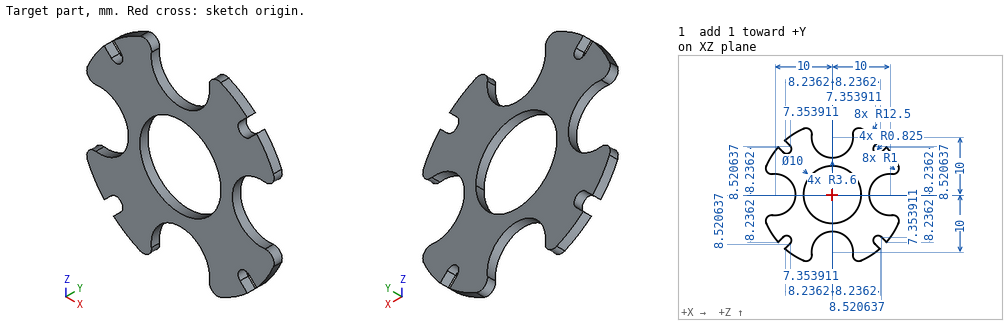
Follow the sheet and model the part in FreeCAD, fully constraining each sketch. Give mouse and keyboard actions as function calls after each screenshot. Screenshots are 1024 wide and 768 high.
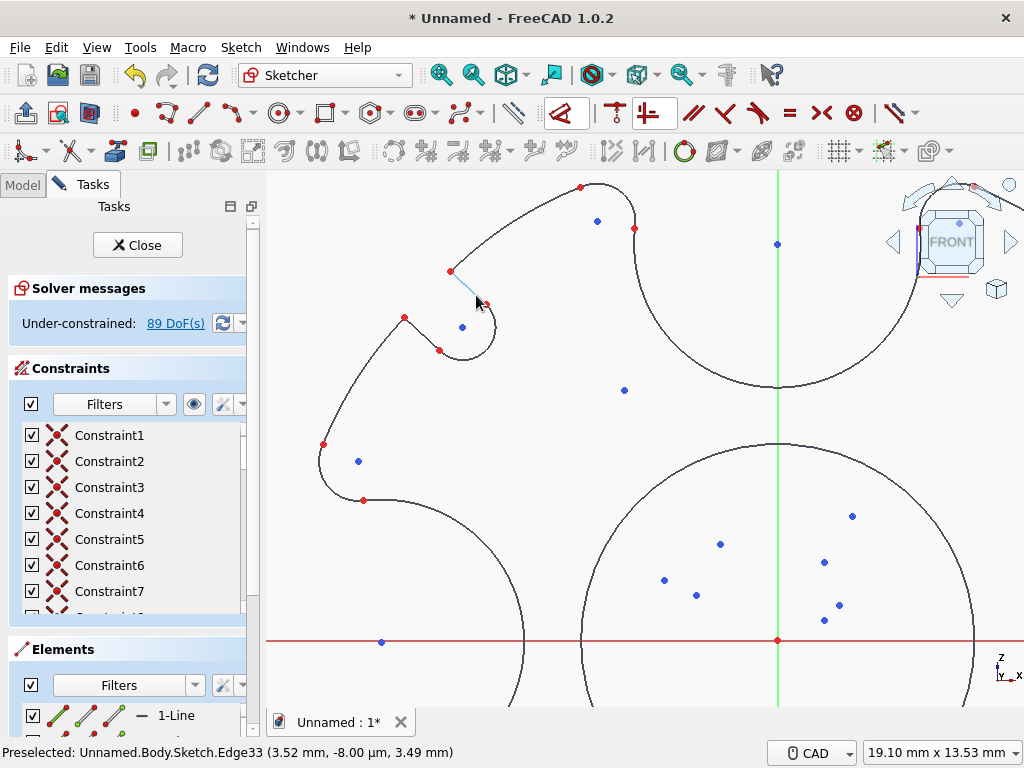
click(475, 295)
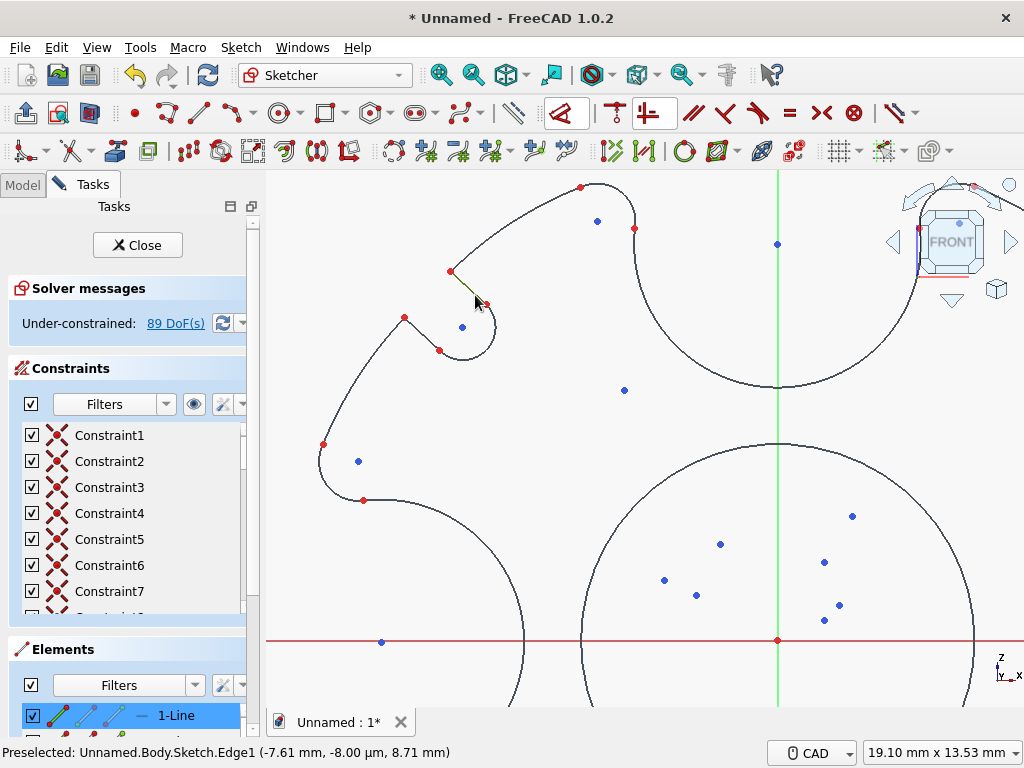
click(468, 360)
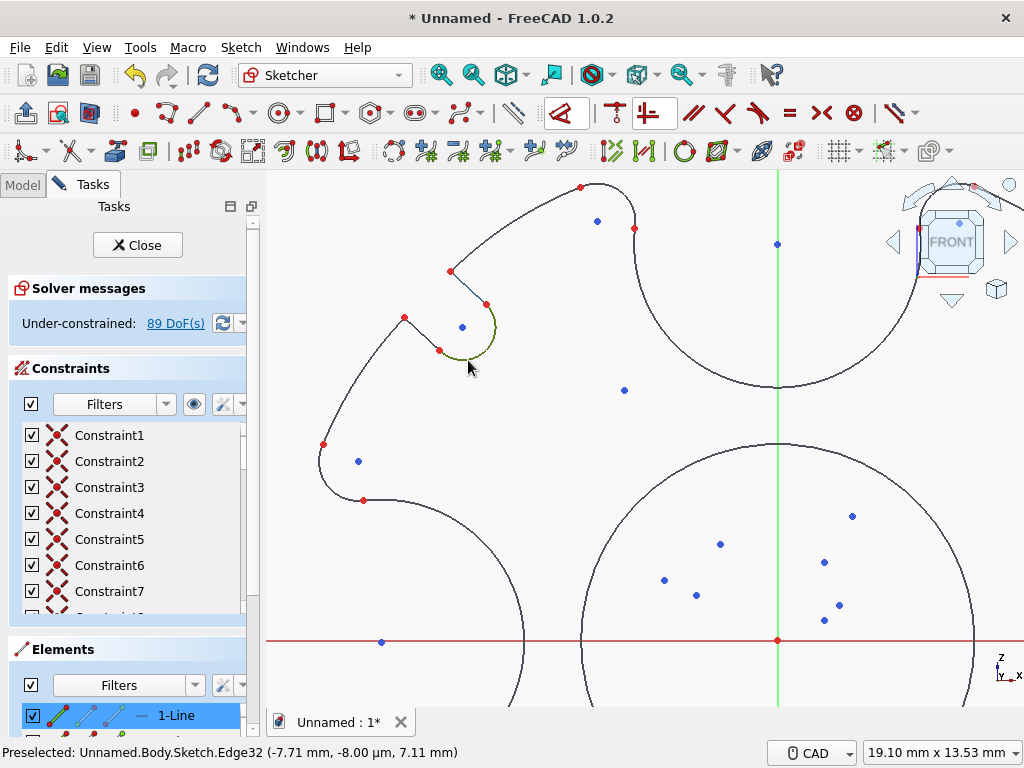
click(758, 114)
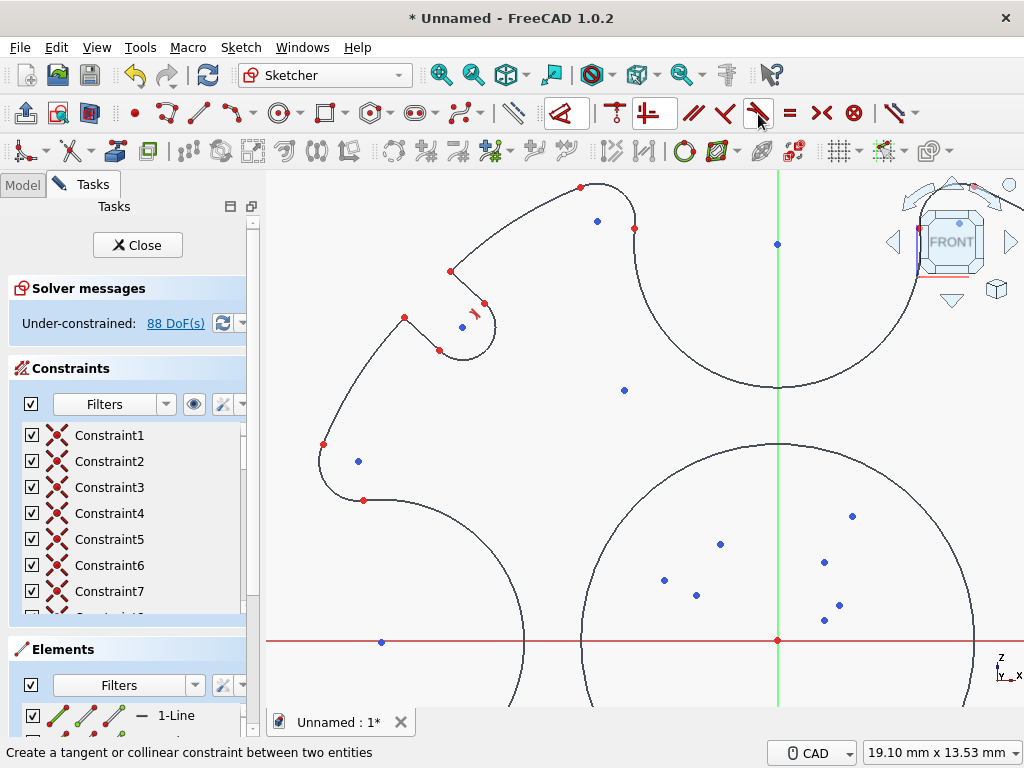
scroll(459, 321, down, 5)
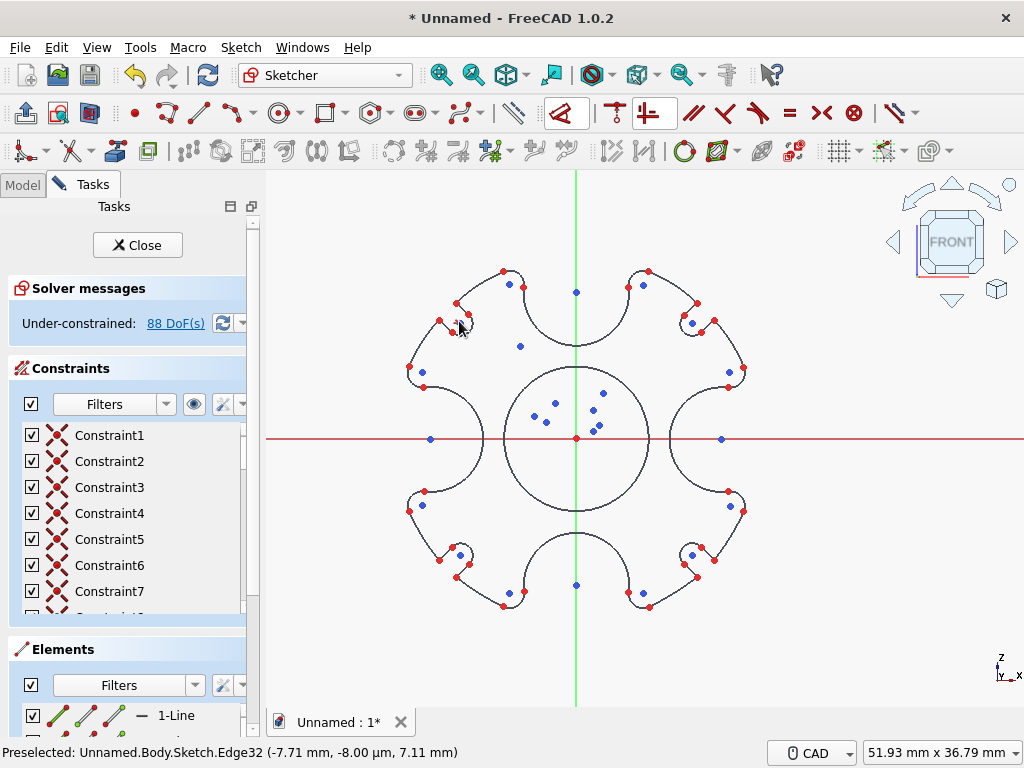
scroll(693, 307, up, 5)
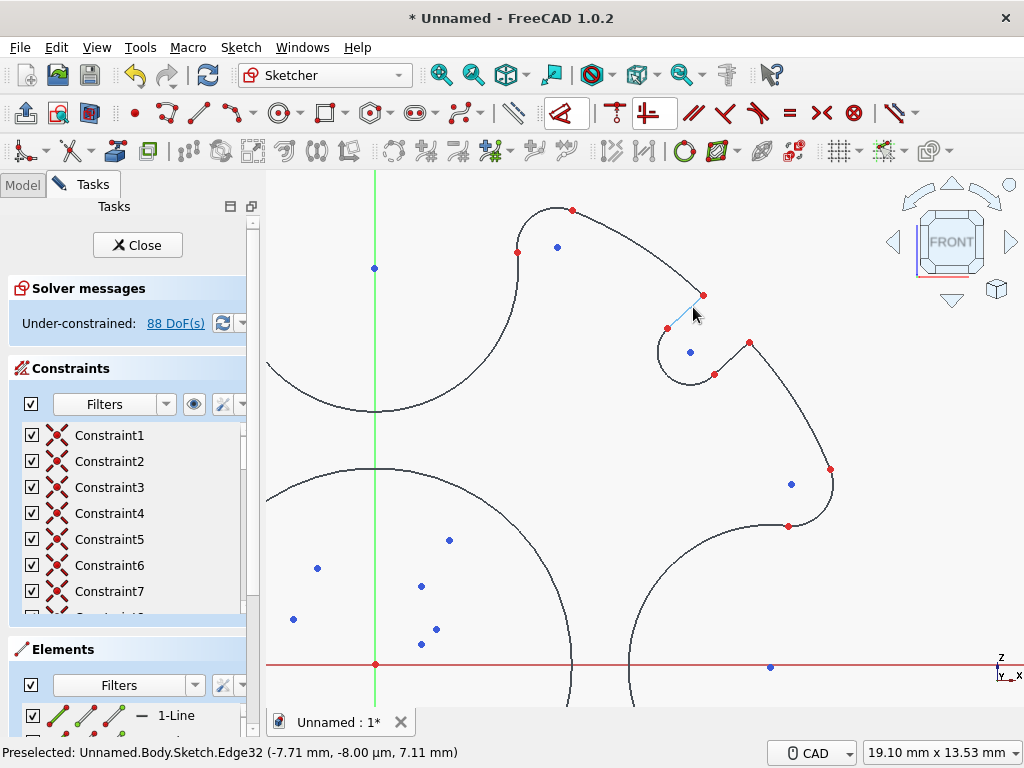
click(693, 306)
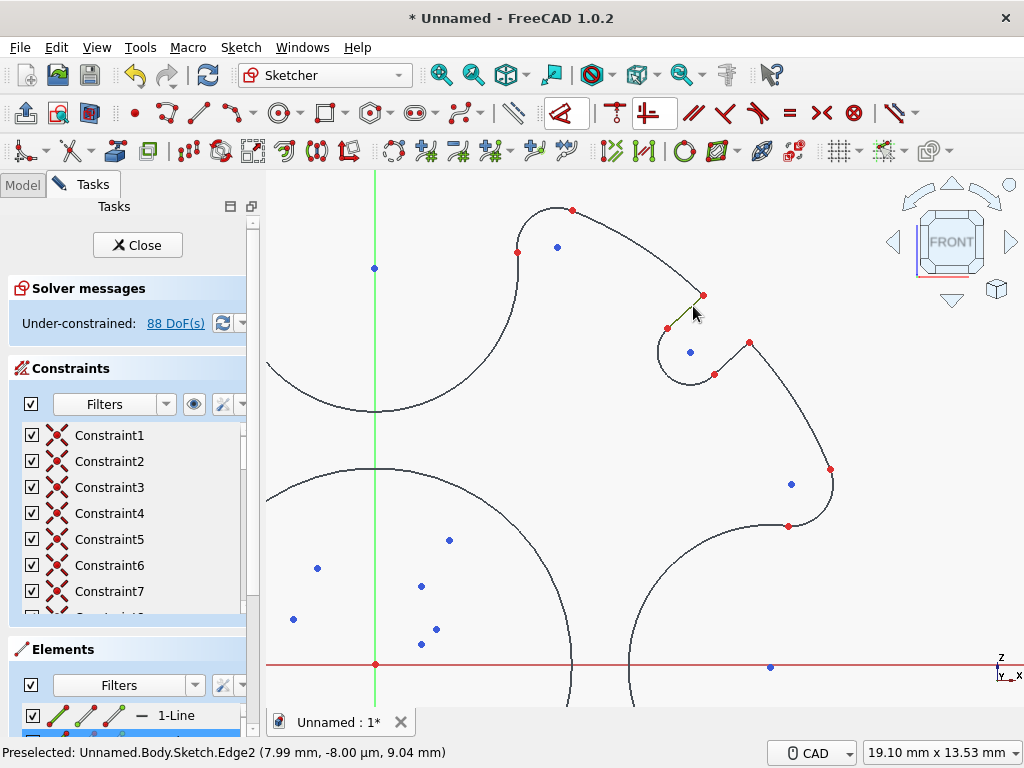
click(658, 357)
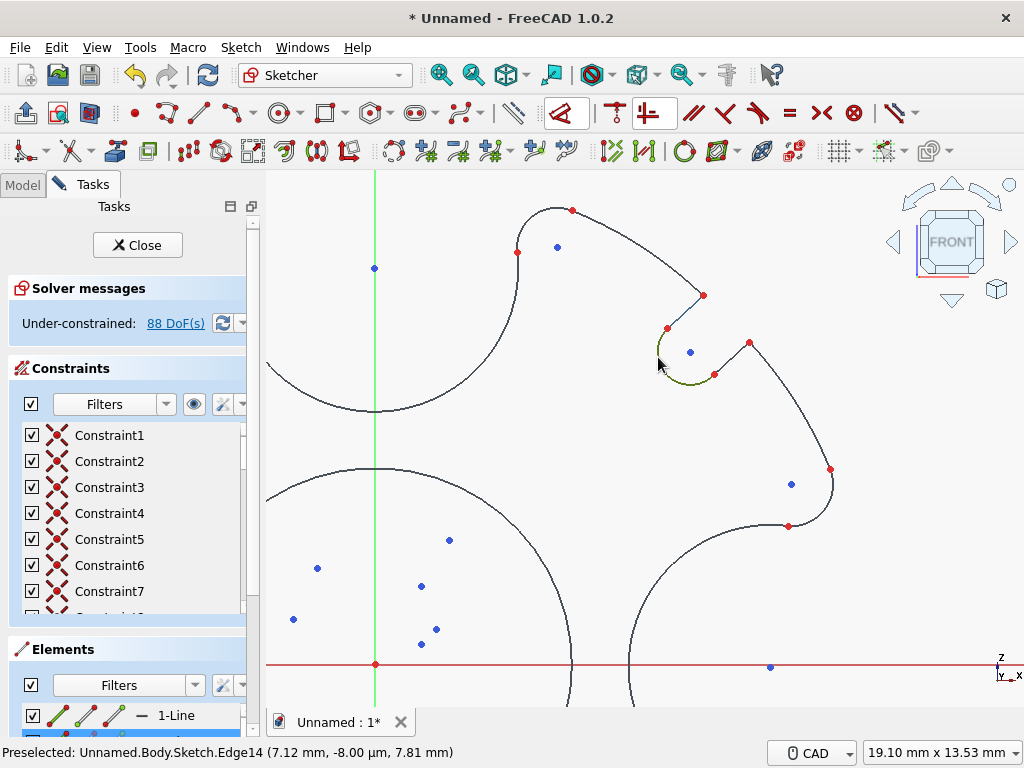
click(758, 114)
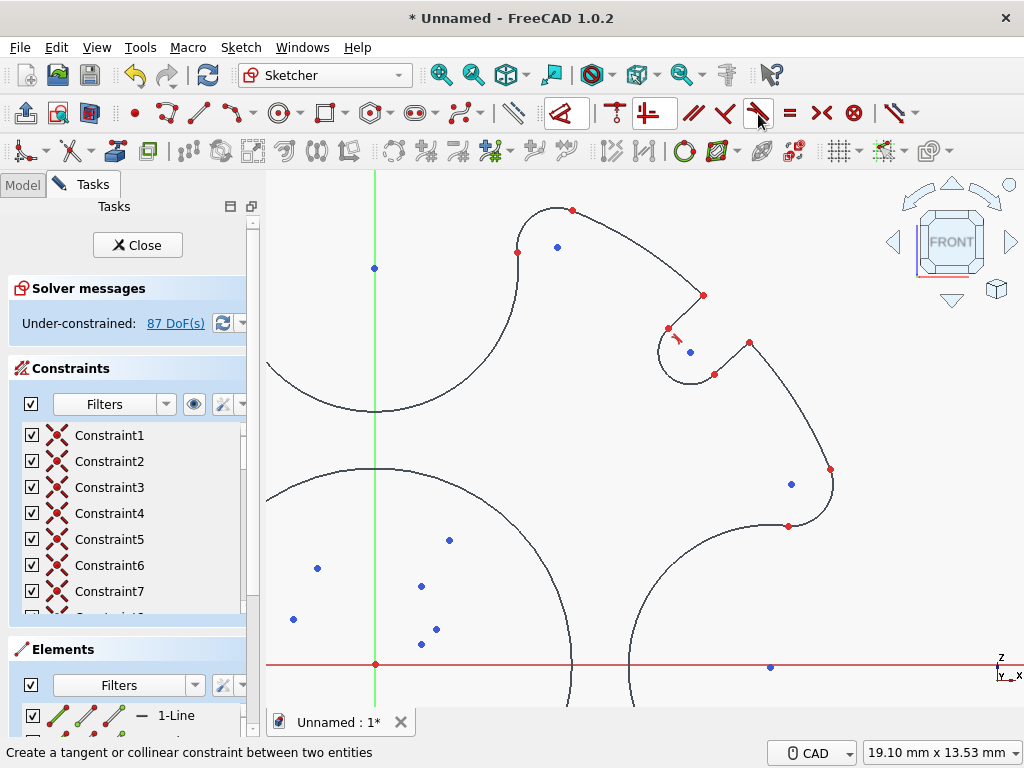
click(725, 365)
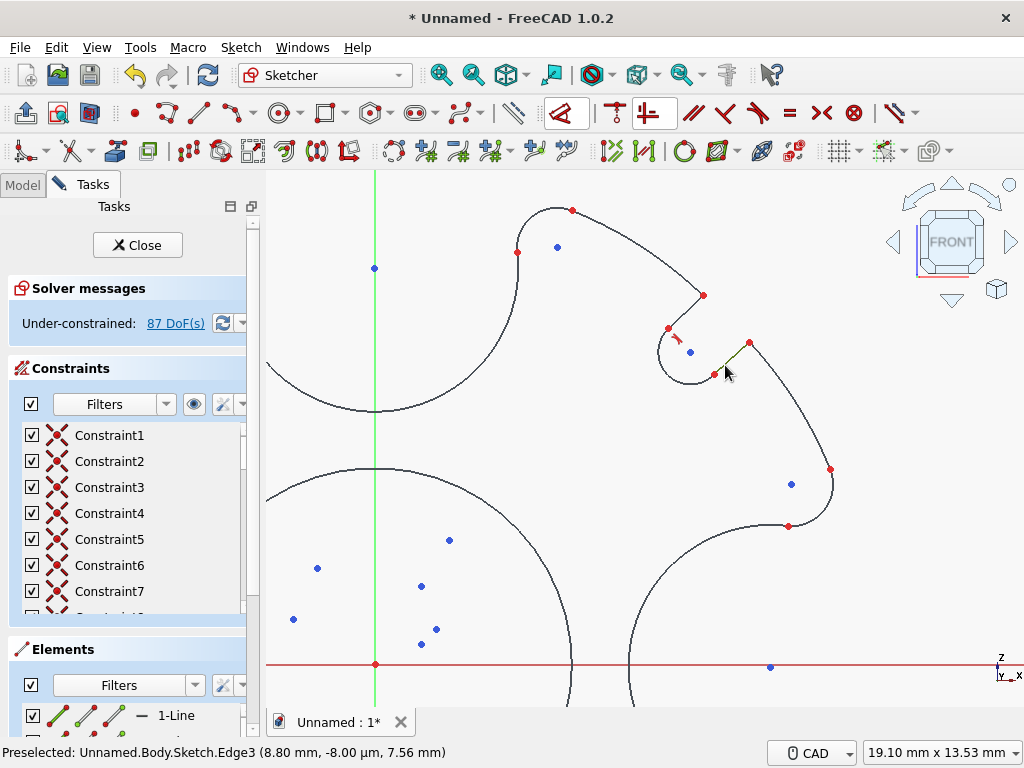
click(659, 357)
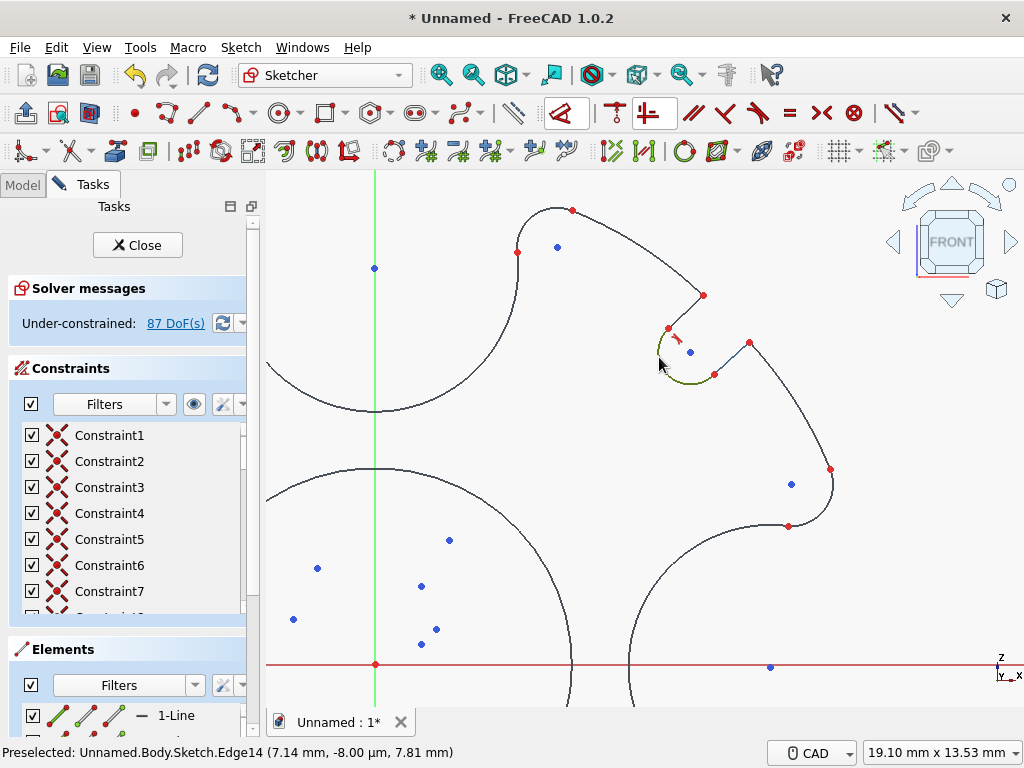
click(758, 114)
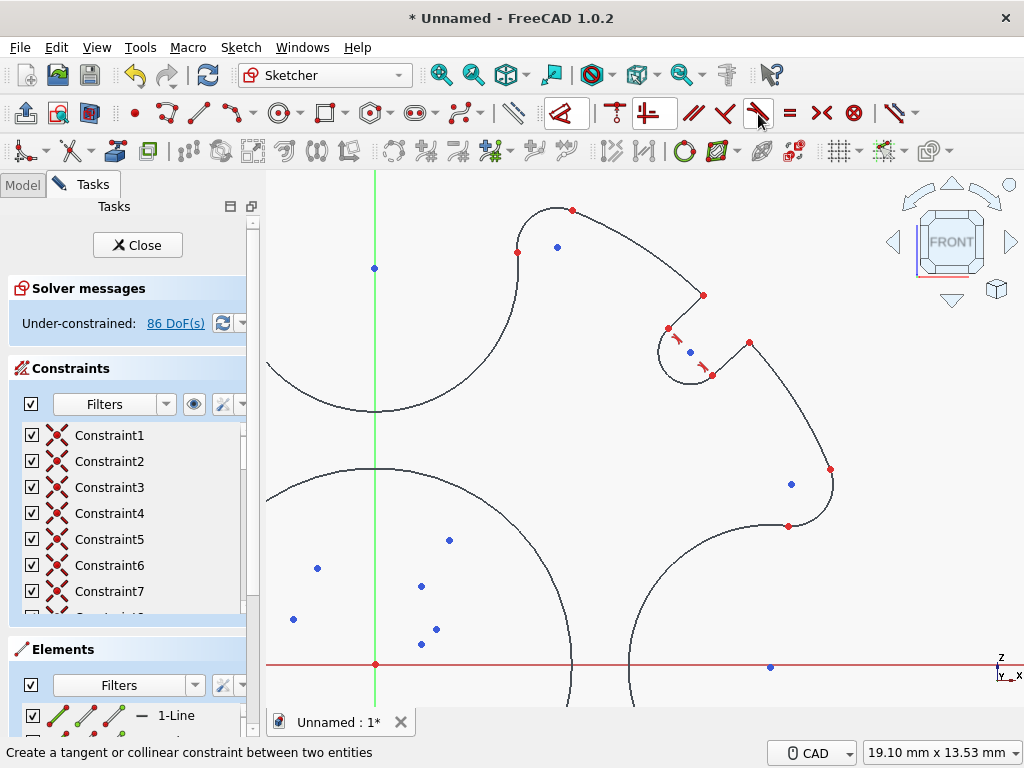
scroll(694, 307, down, 5)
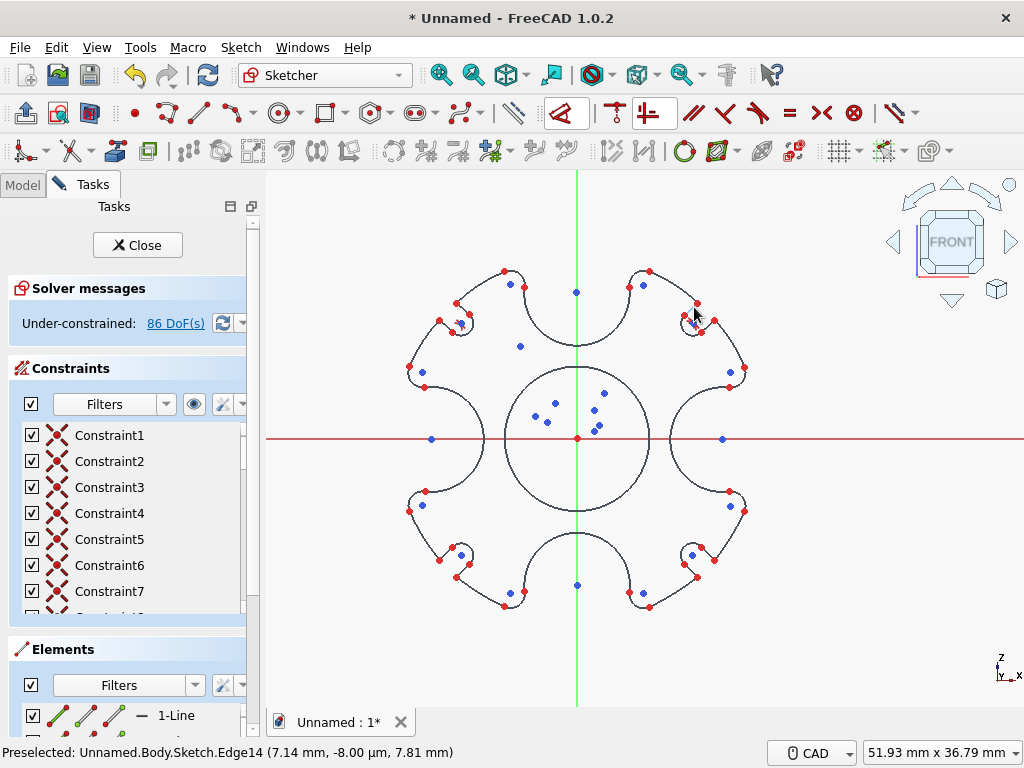
scroll(711, 556, up, 5)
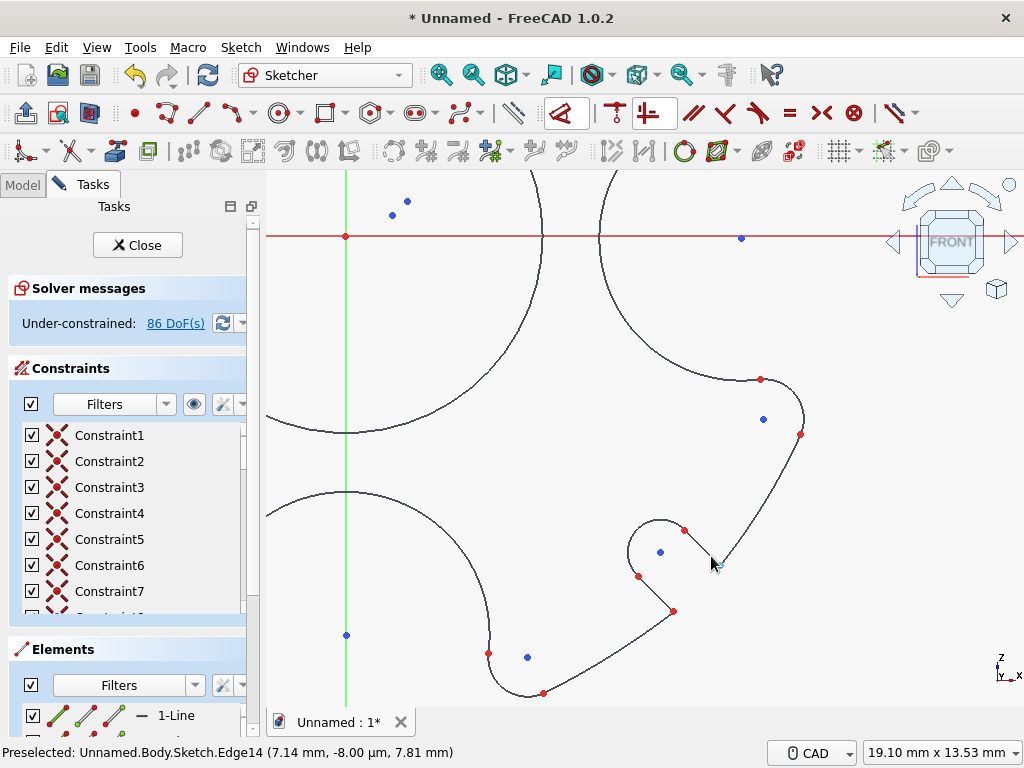
click(710, 555)